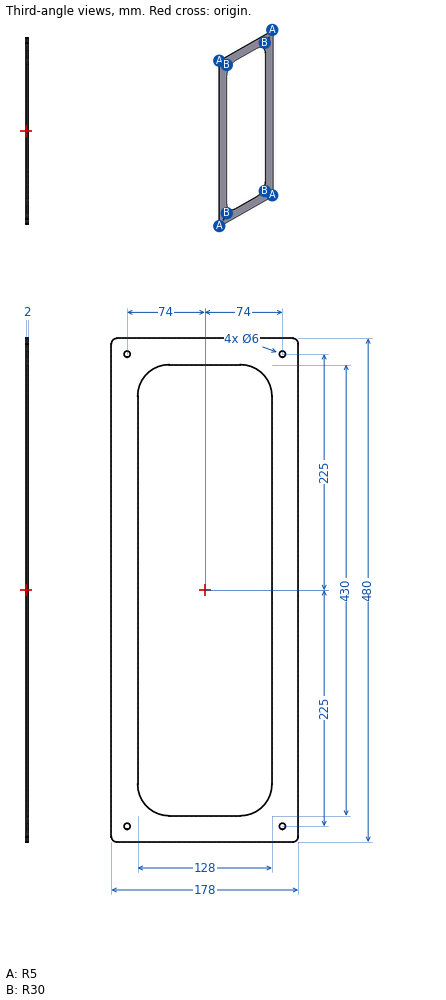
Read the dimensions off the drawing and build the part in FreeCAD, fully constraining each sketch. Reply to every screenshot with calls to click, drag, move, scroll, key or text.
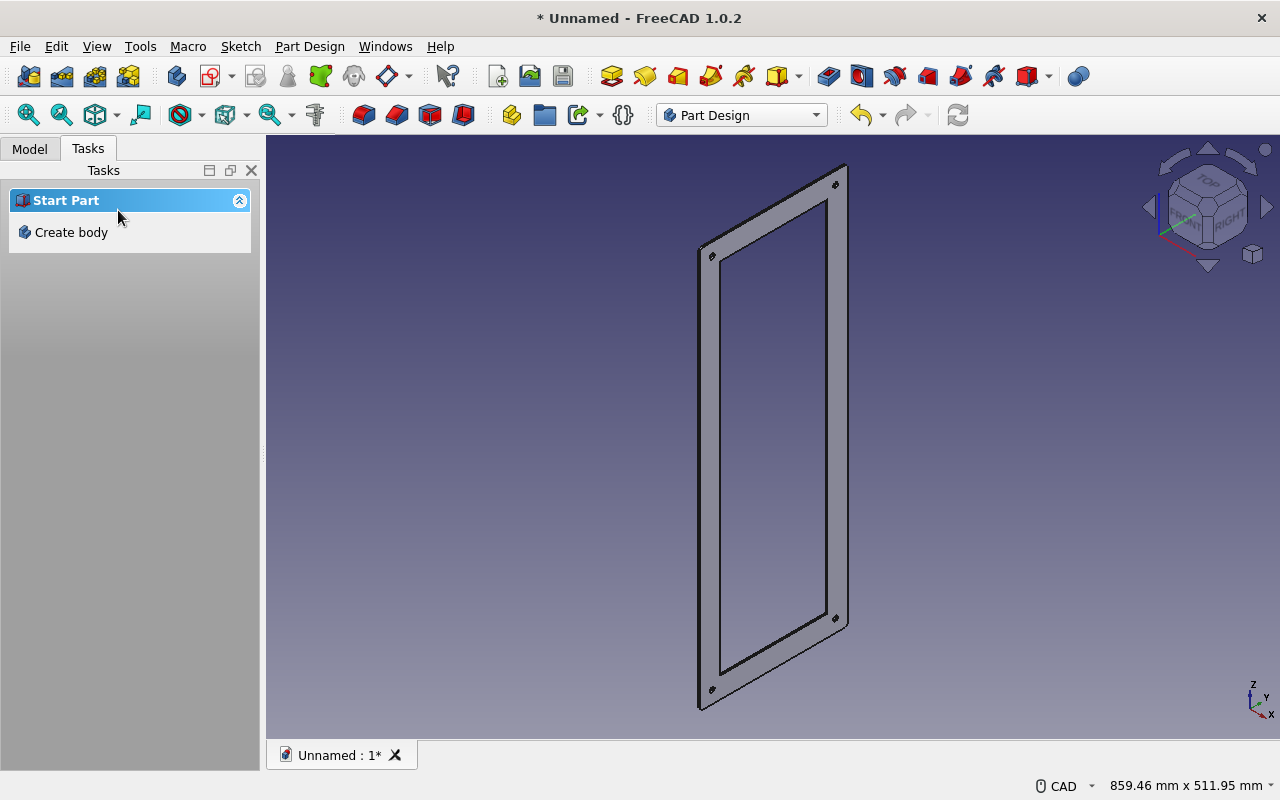
scroll(720, 260, up, 15)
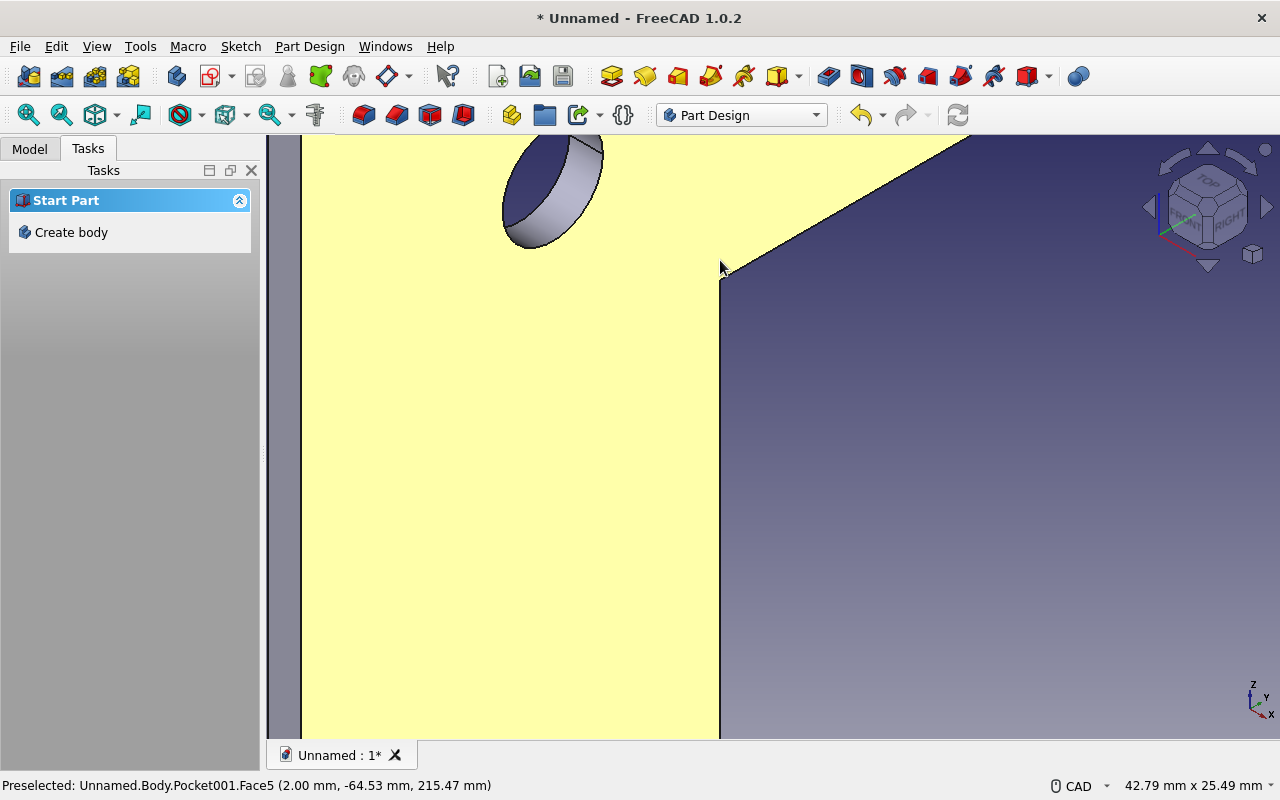
key(v)
key(f)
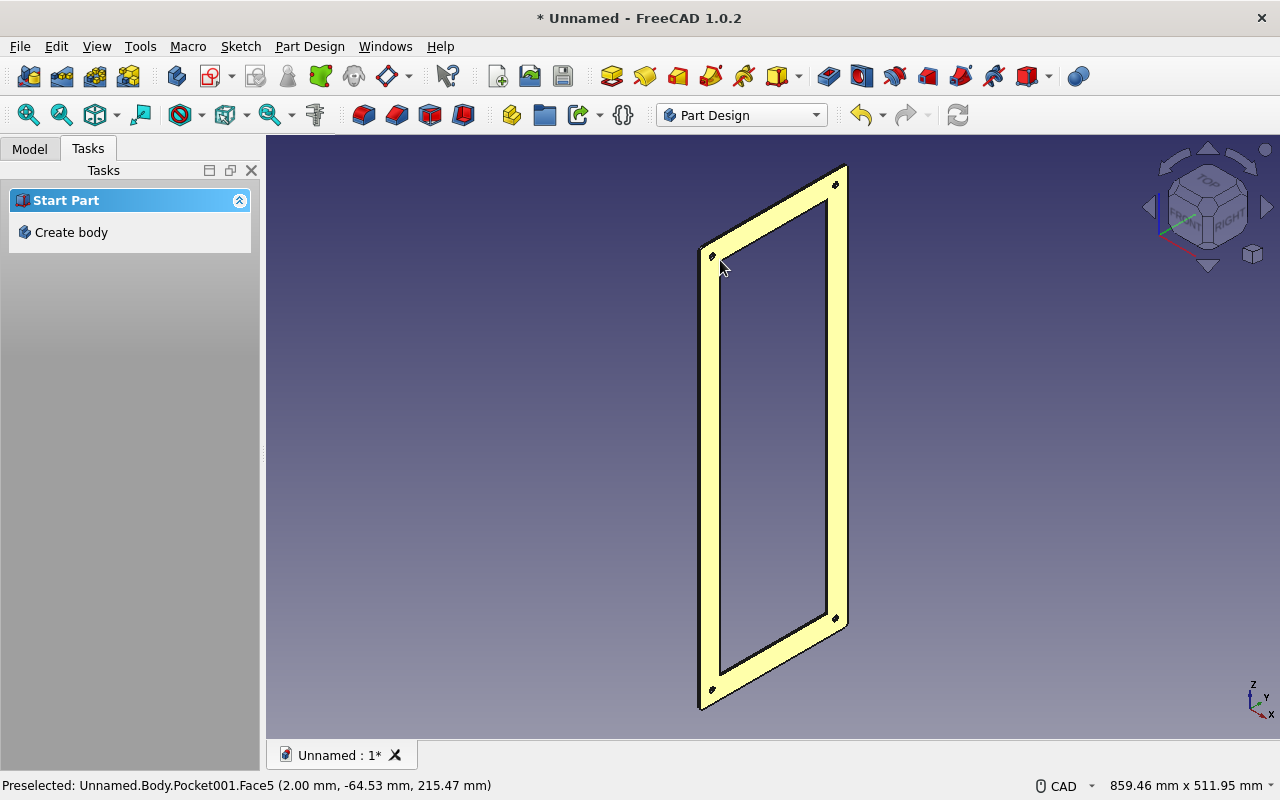
key(2)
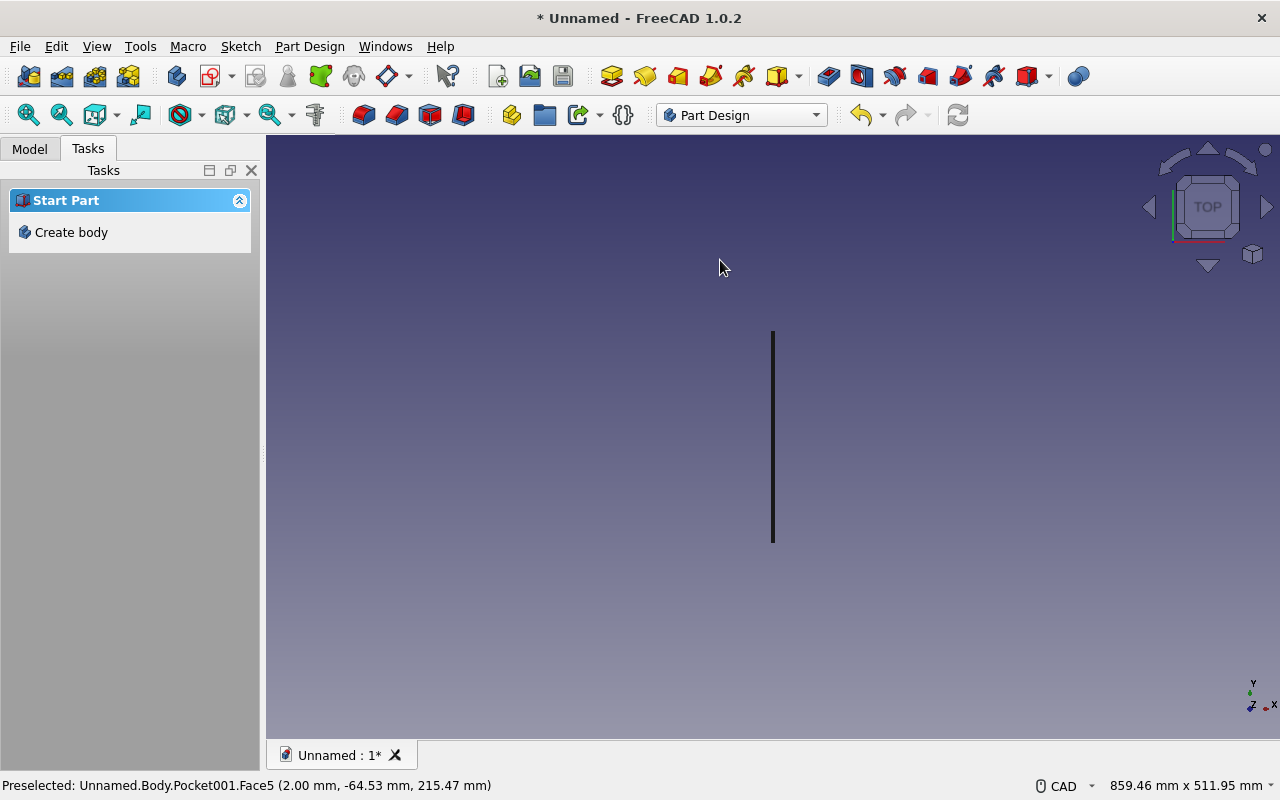
click(29, 116)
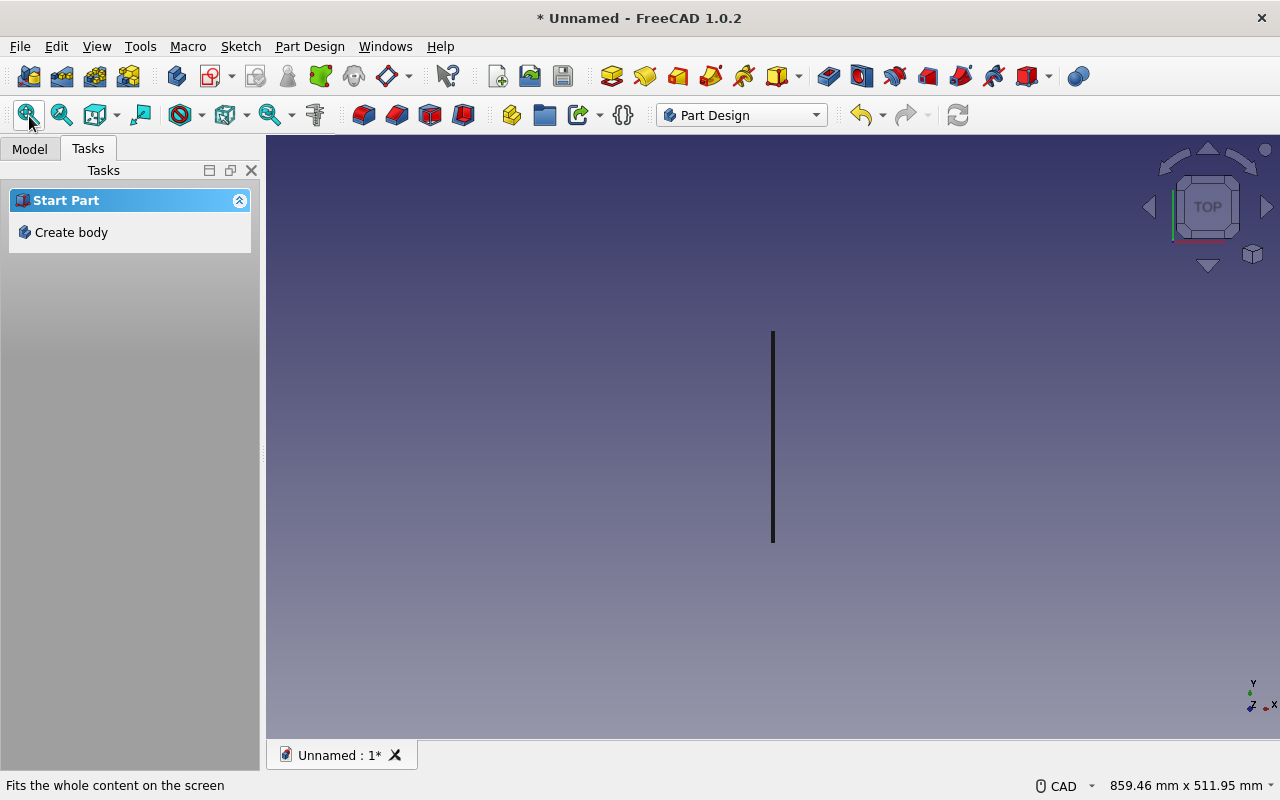
scroll(773, 512, up, 15)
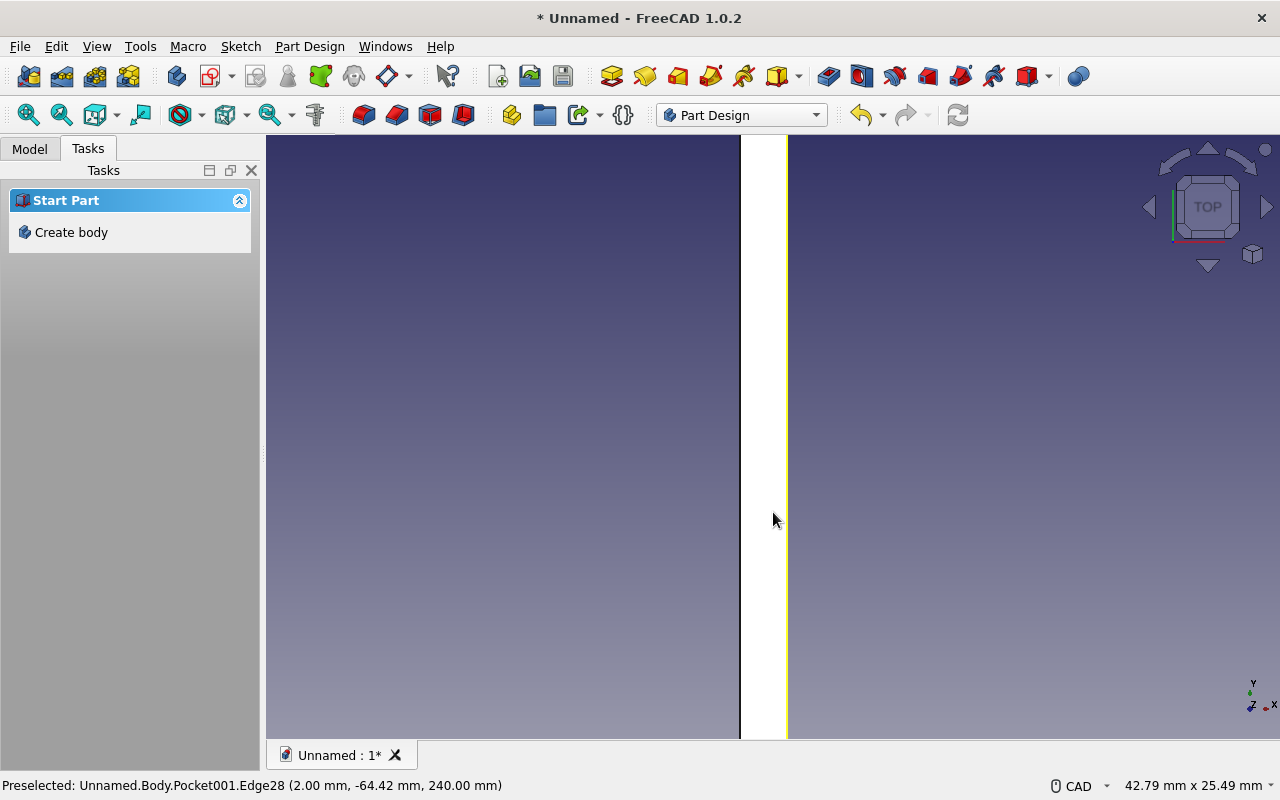
key(v)
key(f)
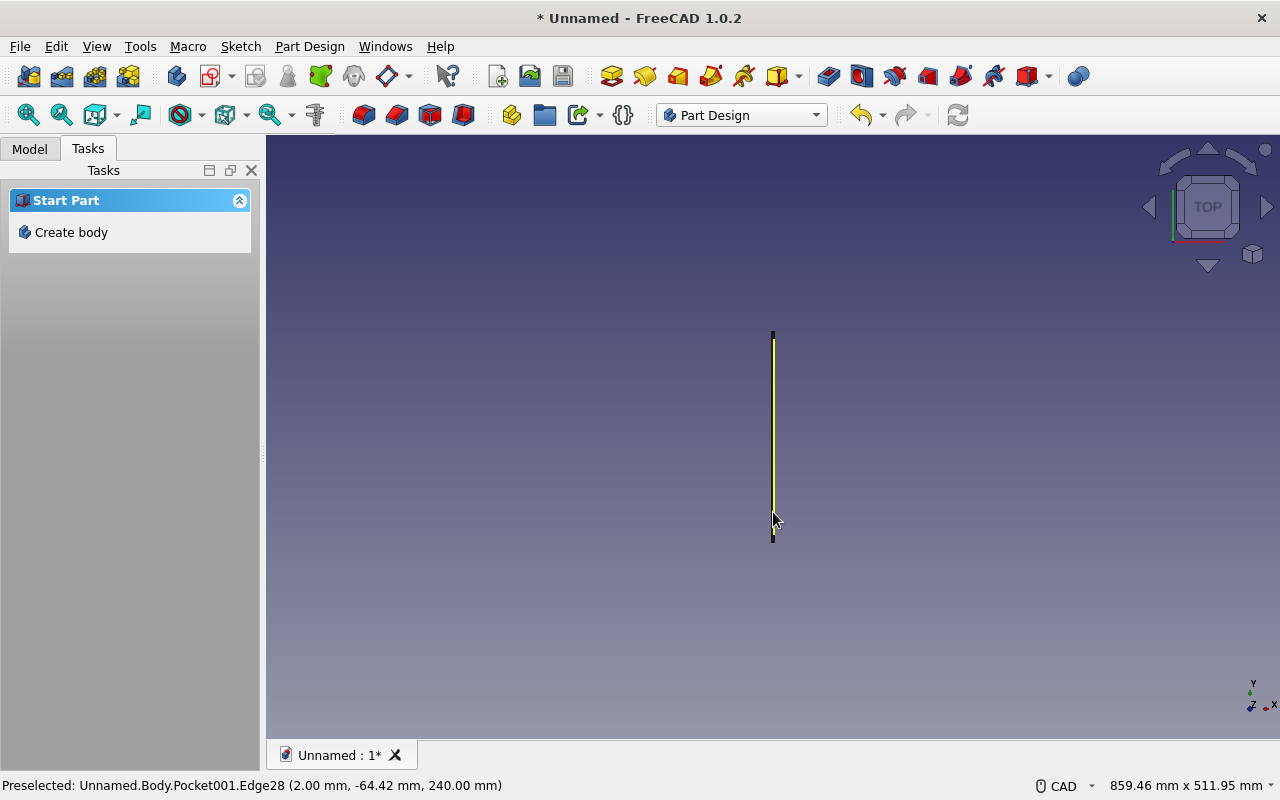
key(0)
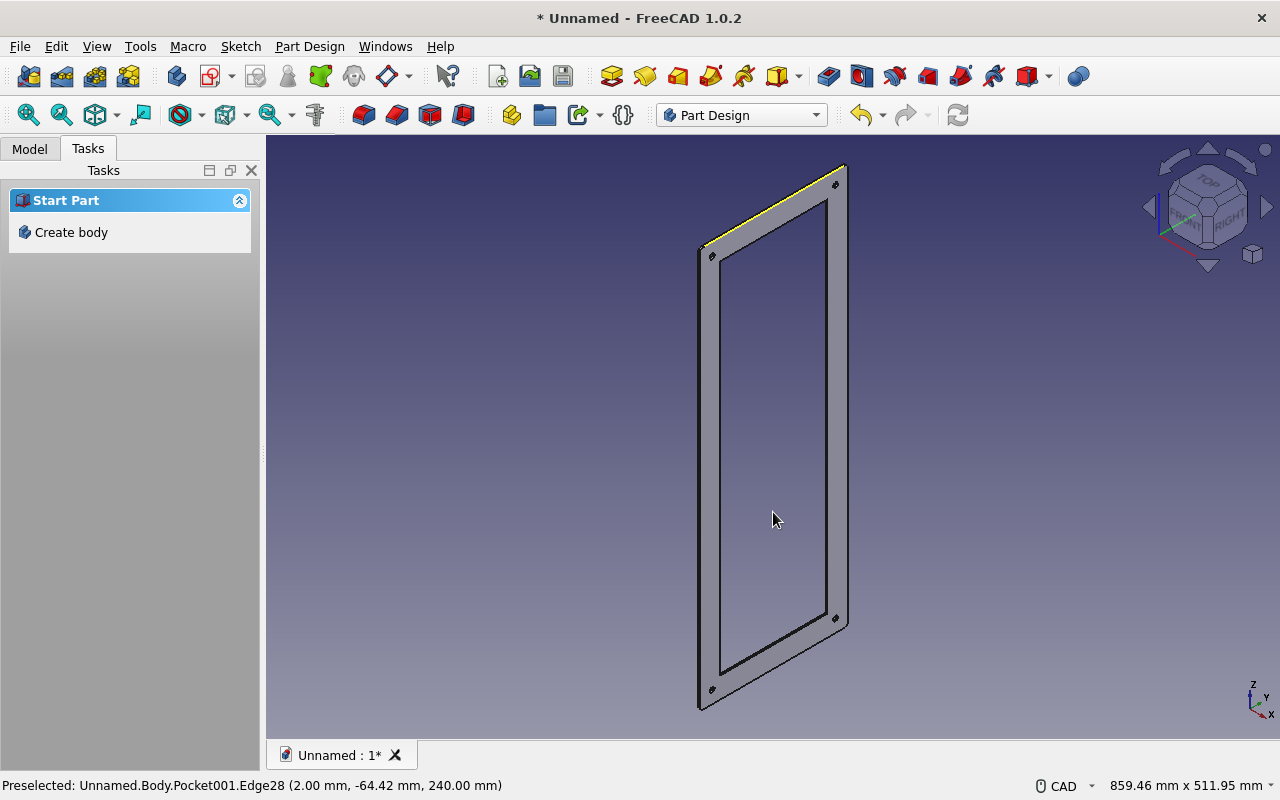
scroll(720, 260, up, 15)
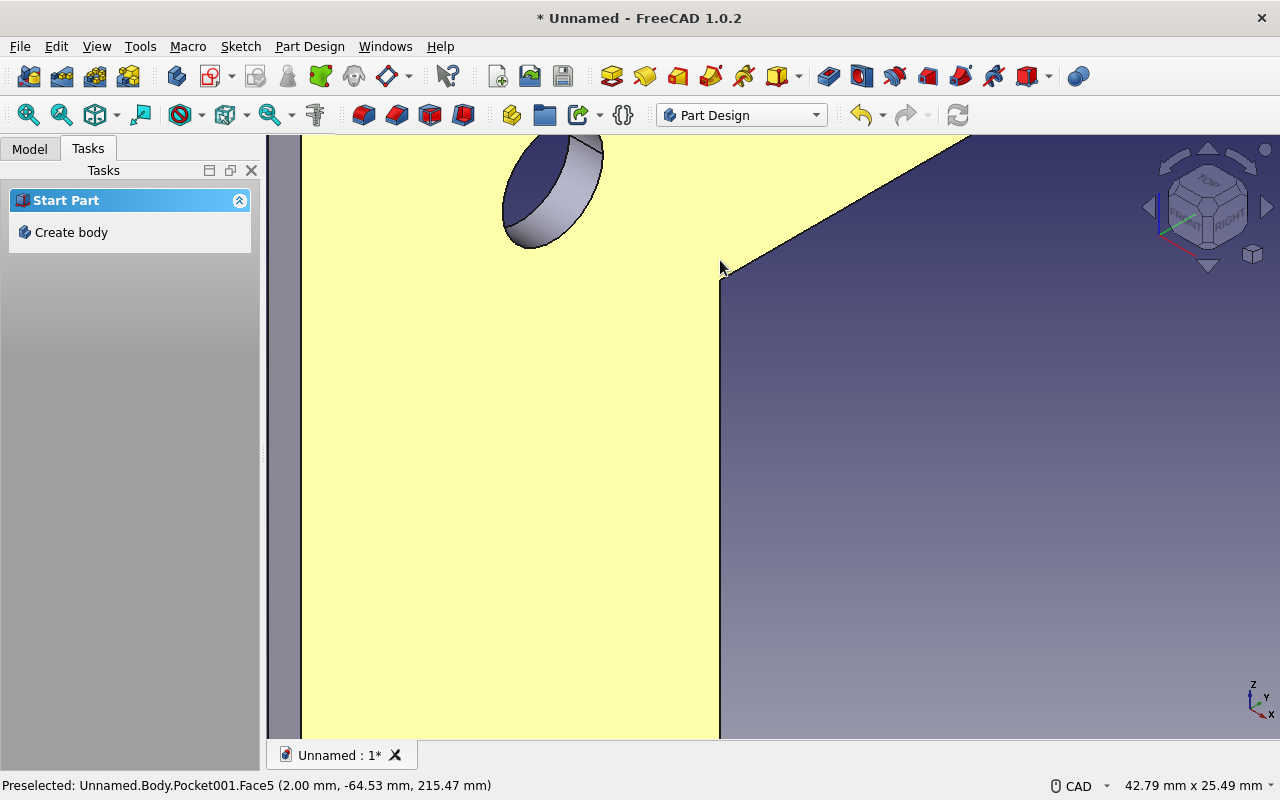
key(v)
key(f)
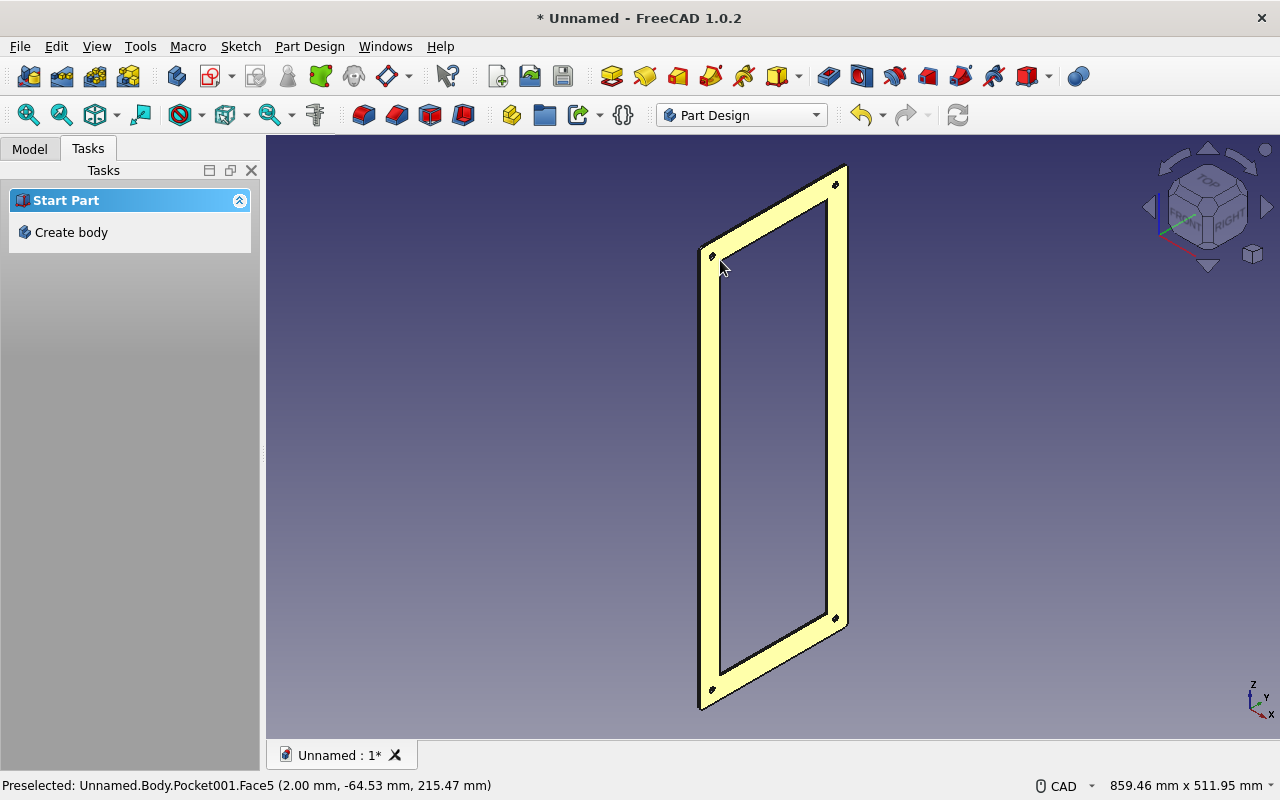
key(1)